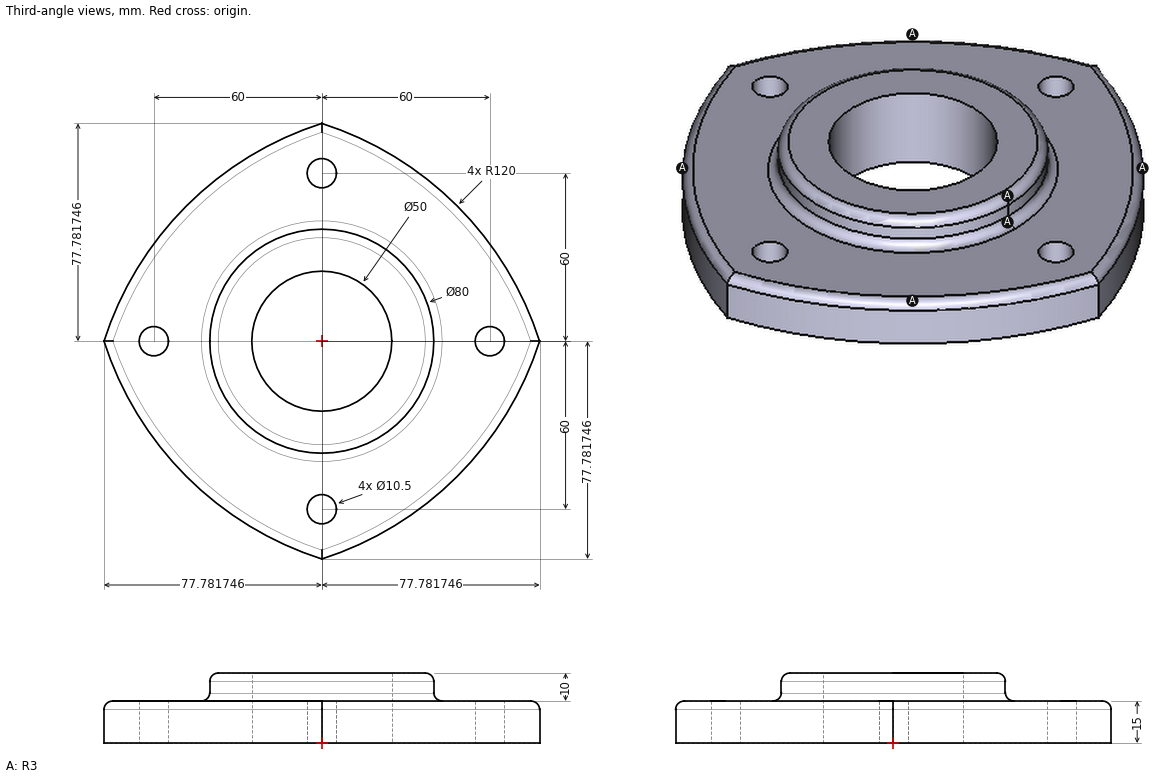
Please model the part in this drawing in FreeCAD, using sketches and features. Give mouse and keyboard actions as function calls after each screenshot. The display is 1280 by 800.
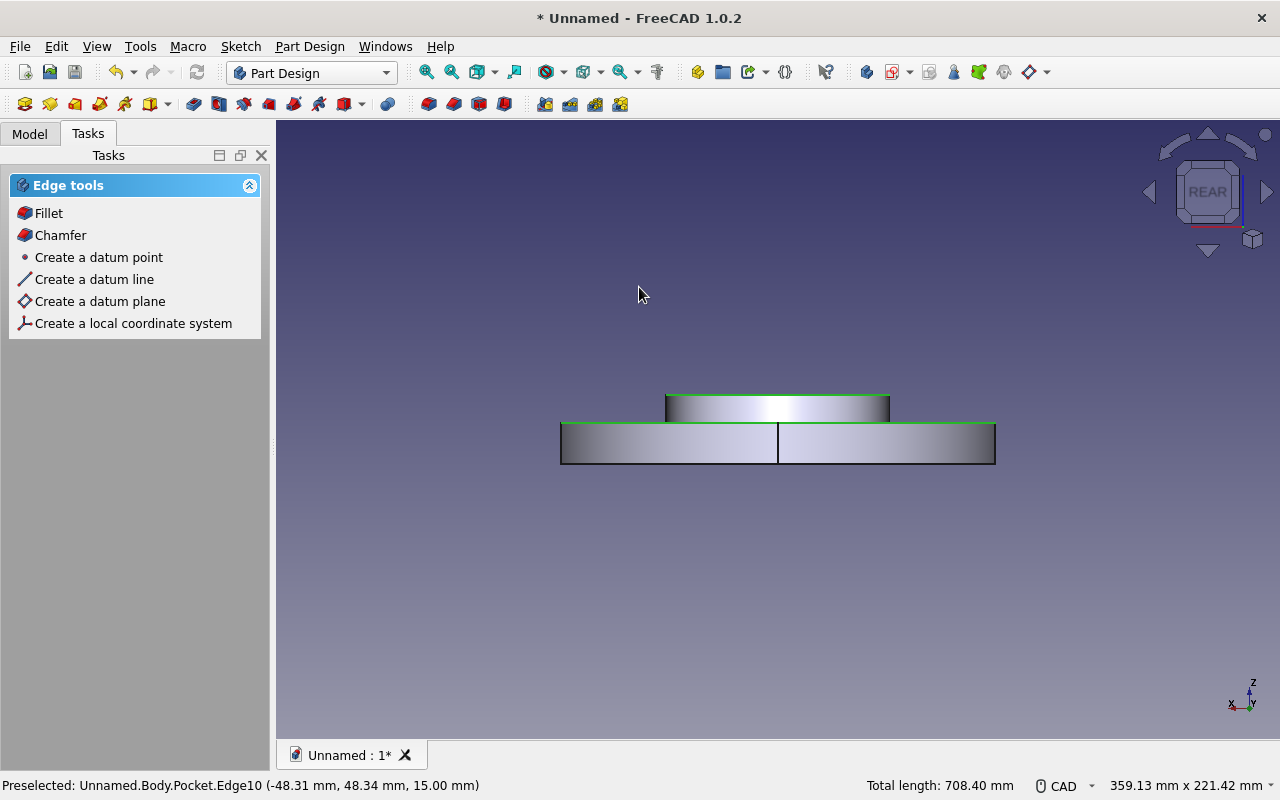
key(6)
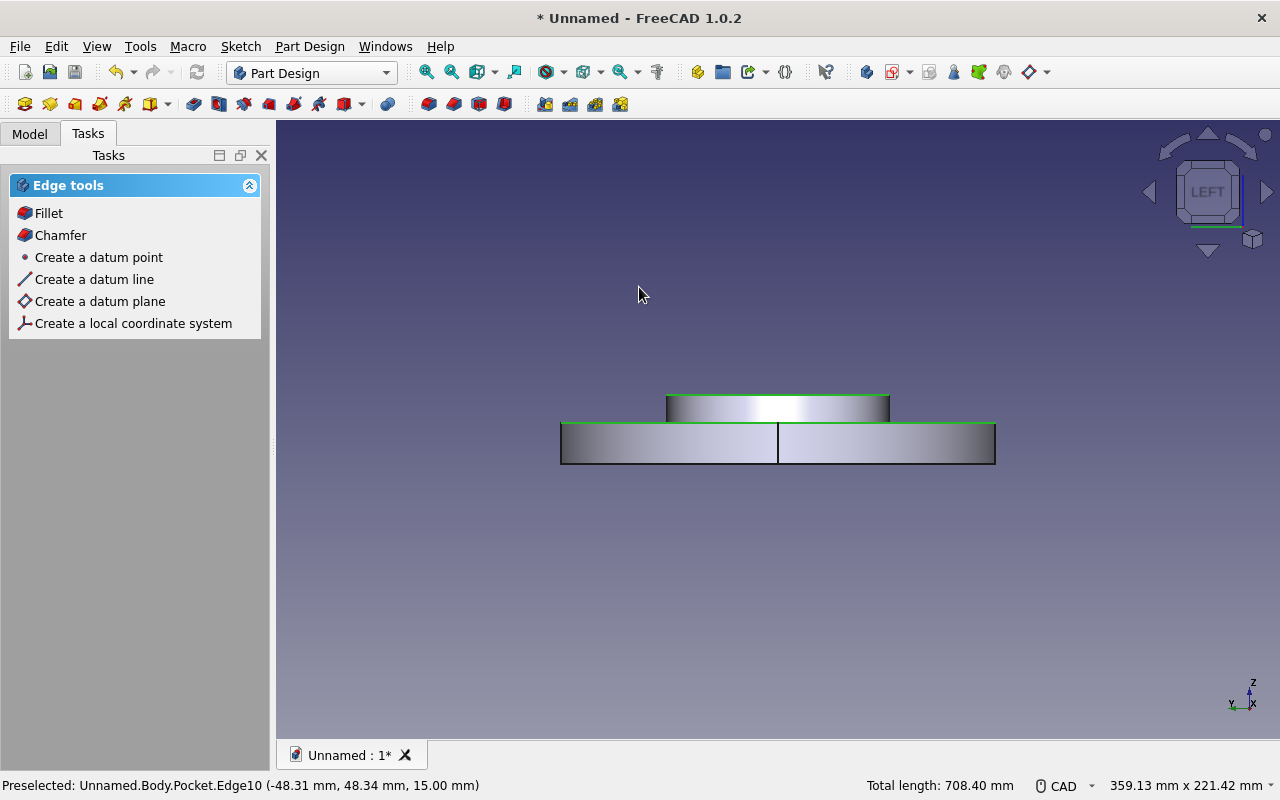
key(v)
key(f)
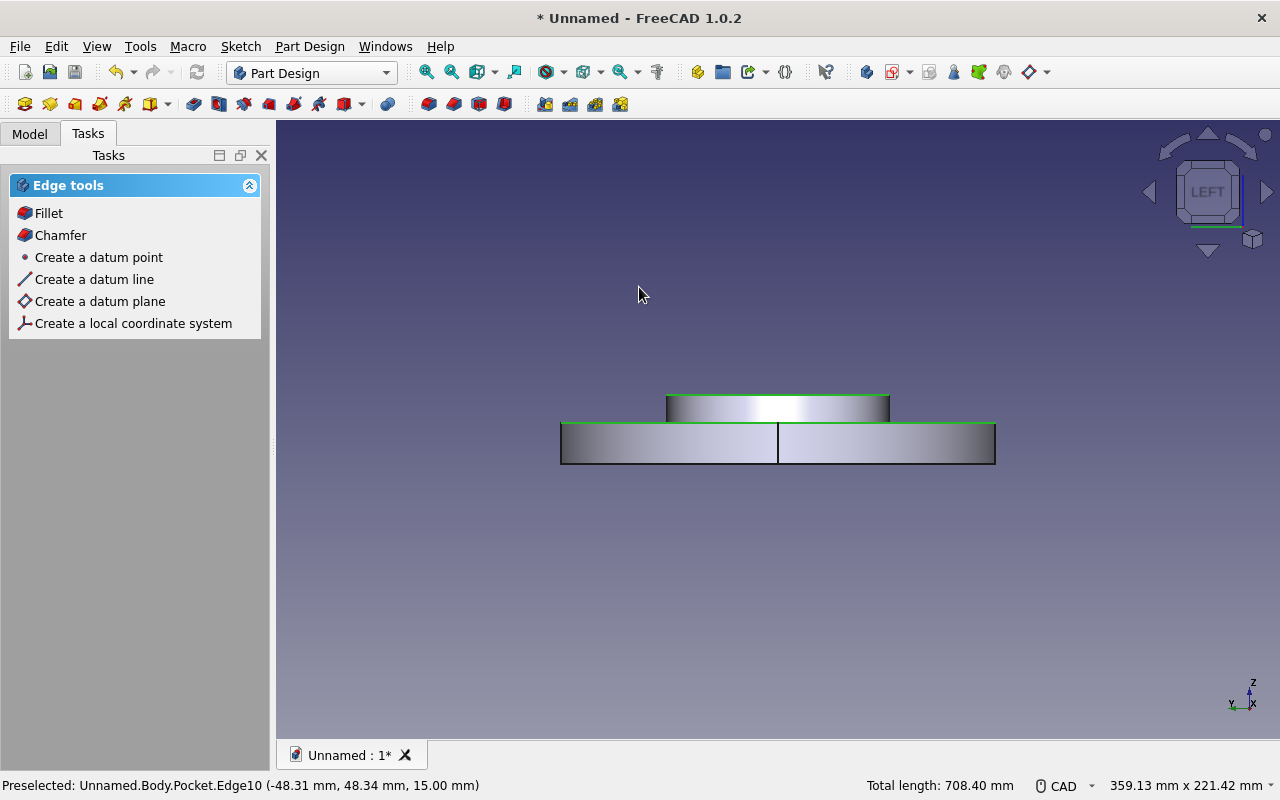
key(v)
key(3)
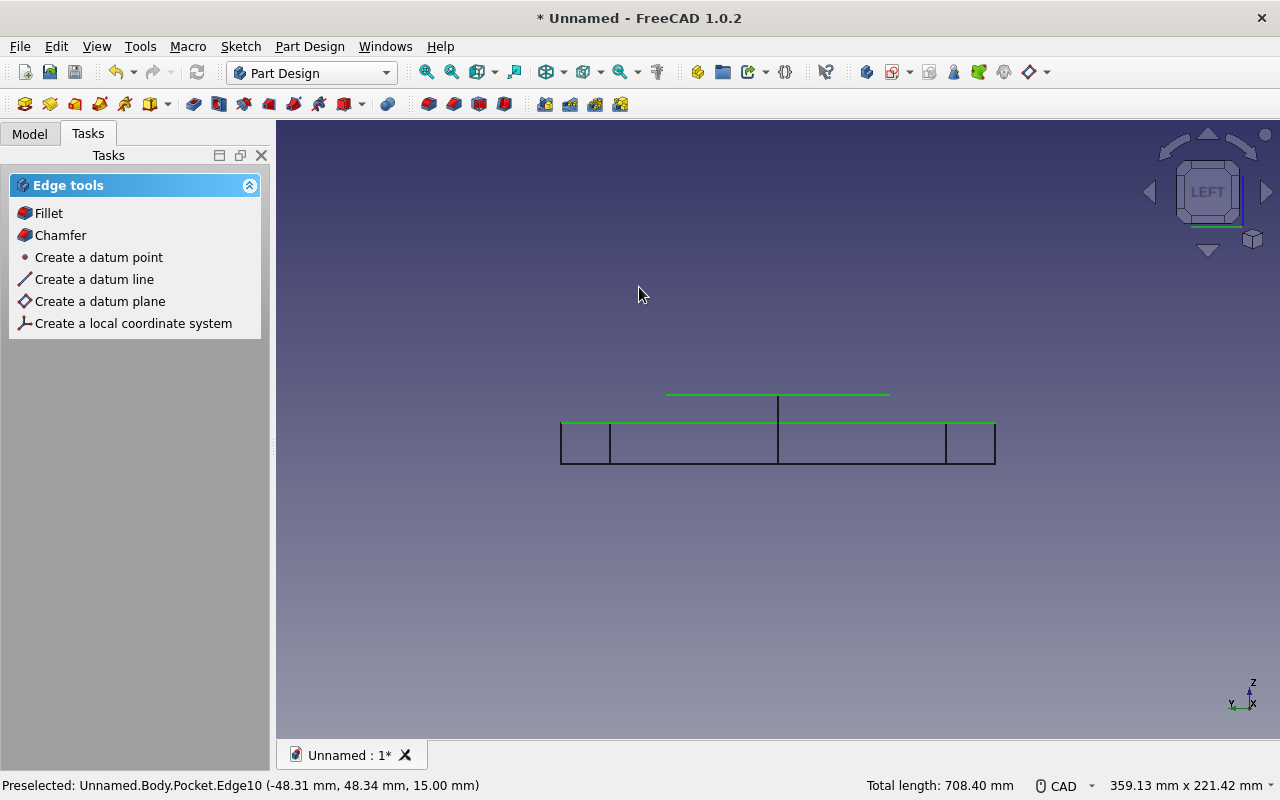
key(0)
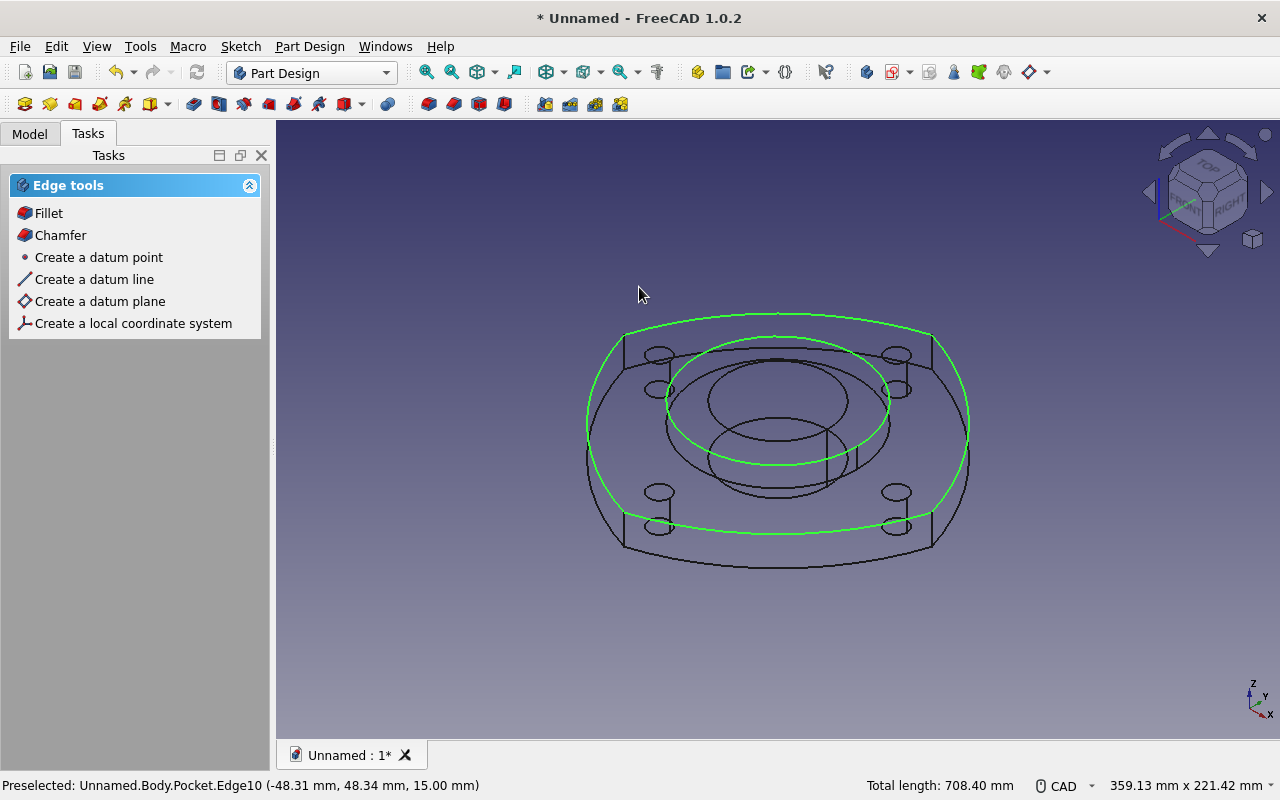
click(699, 377, ctrl)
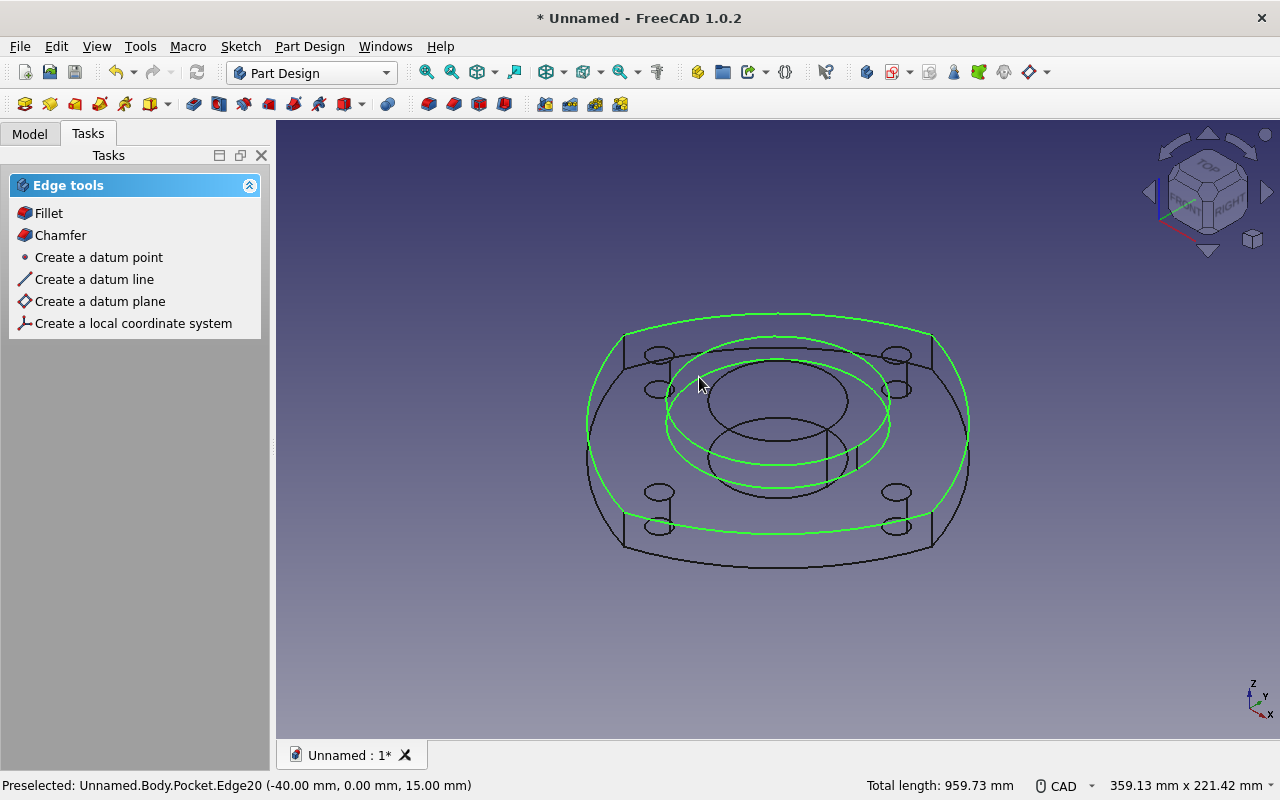
key(v)
key(1)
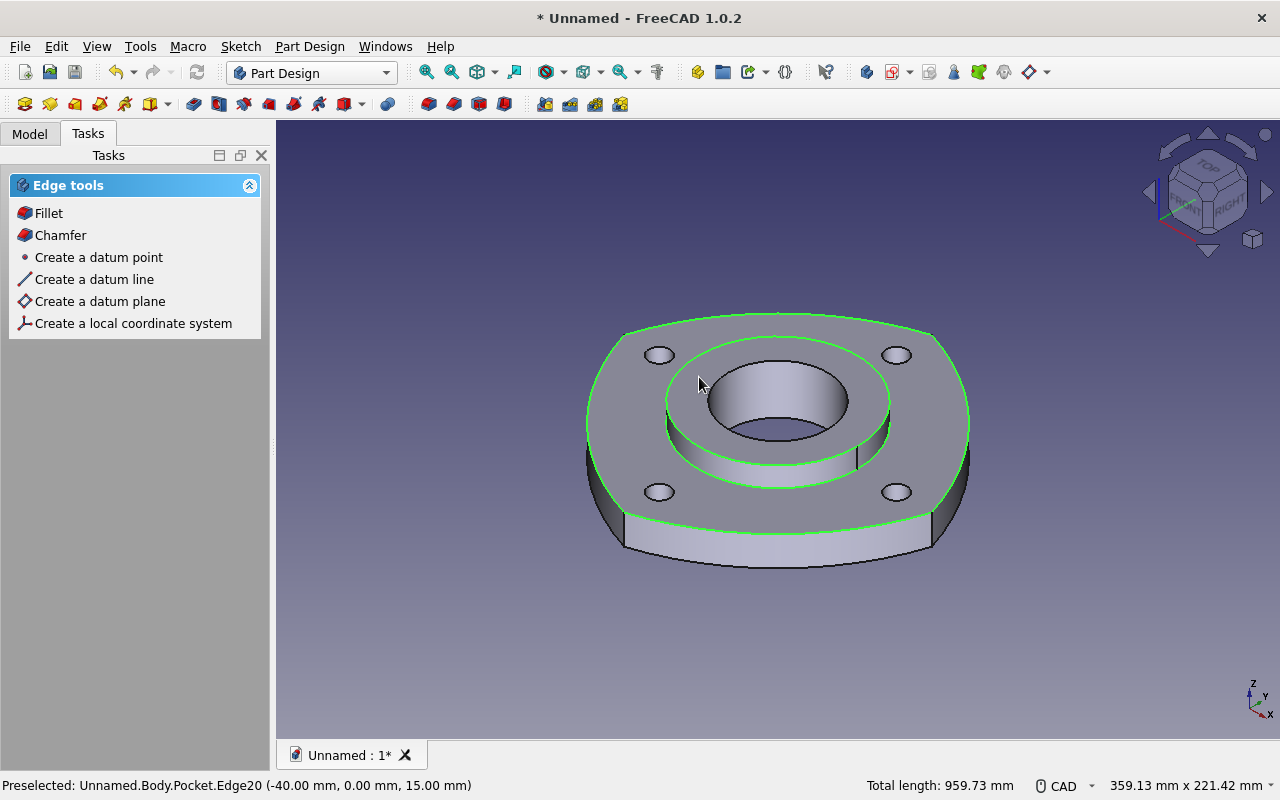
click(429, 104)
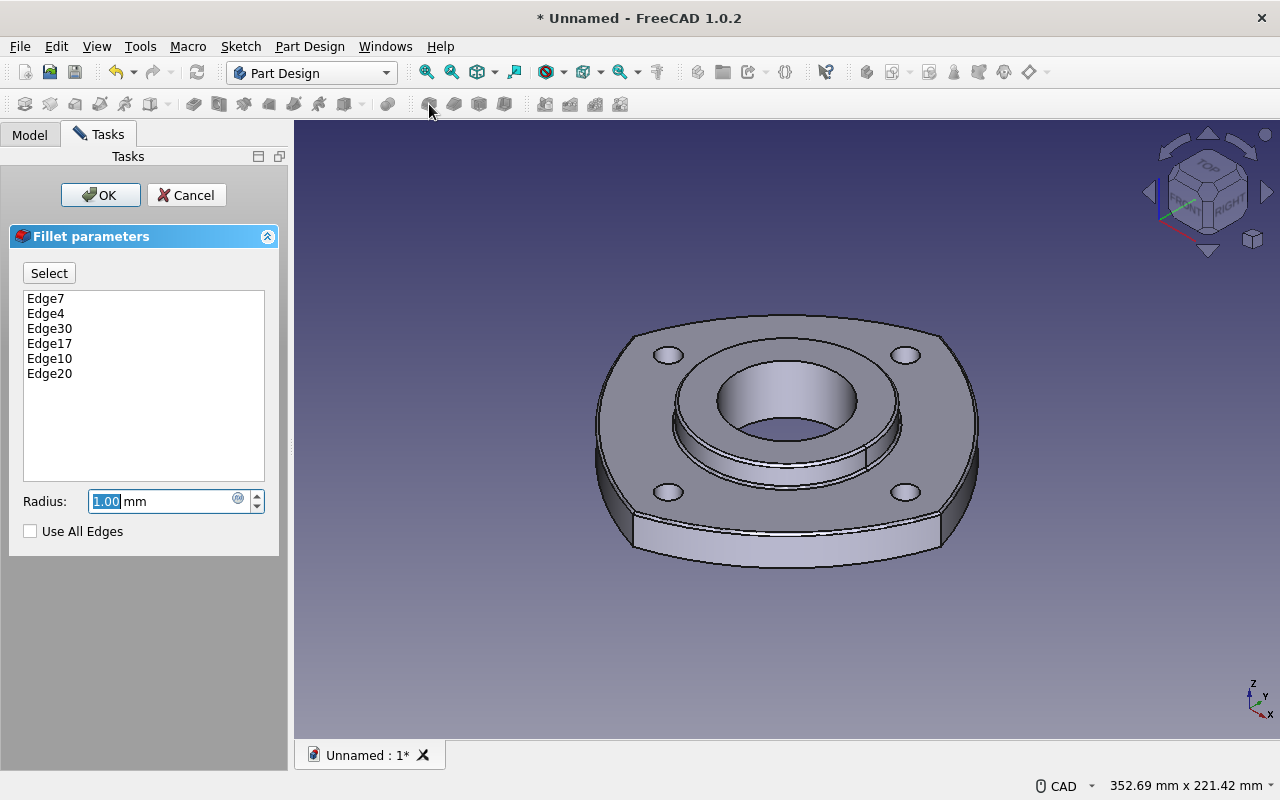
text(3)
key(Tab)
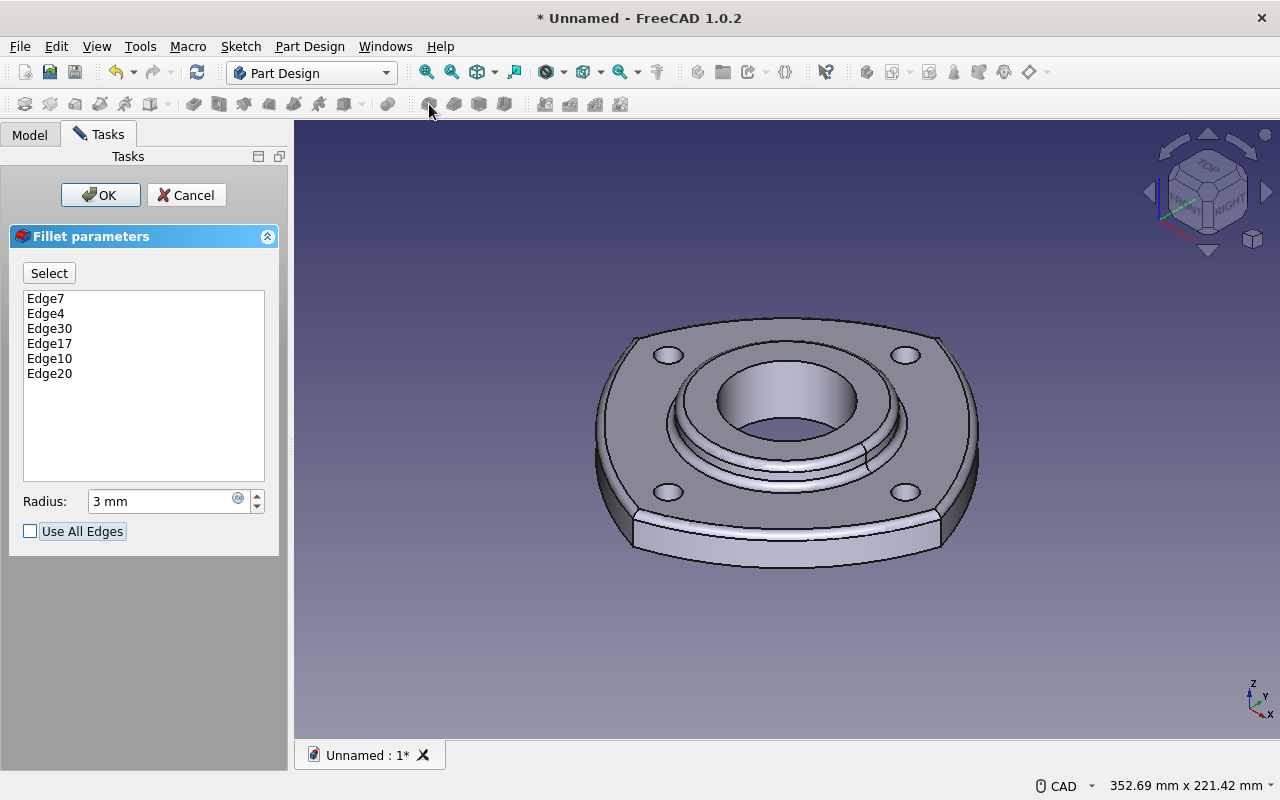
click(101, 195)